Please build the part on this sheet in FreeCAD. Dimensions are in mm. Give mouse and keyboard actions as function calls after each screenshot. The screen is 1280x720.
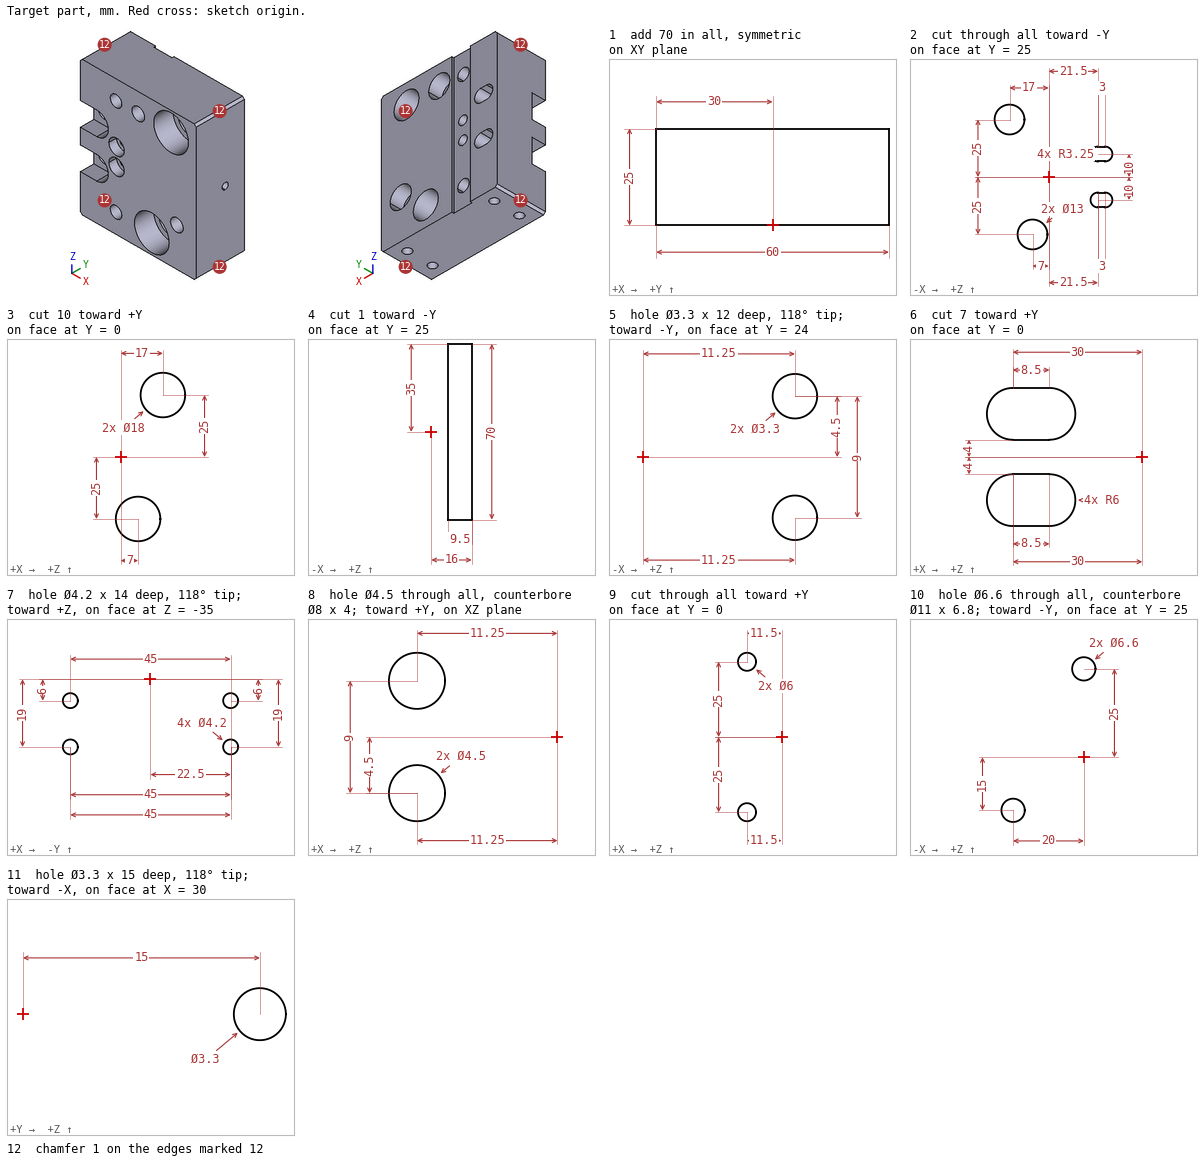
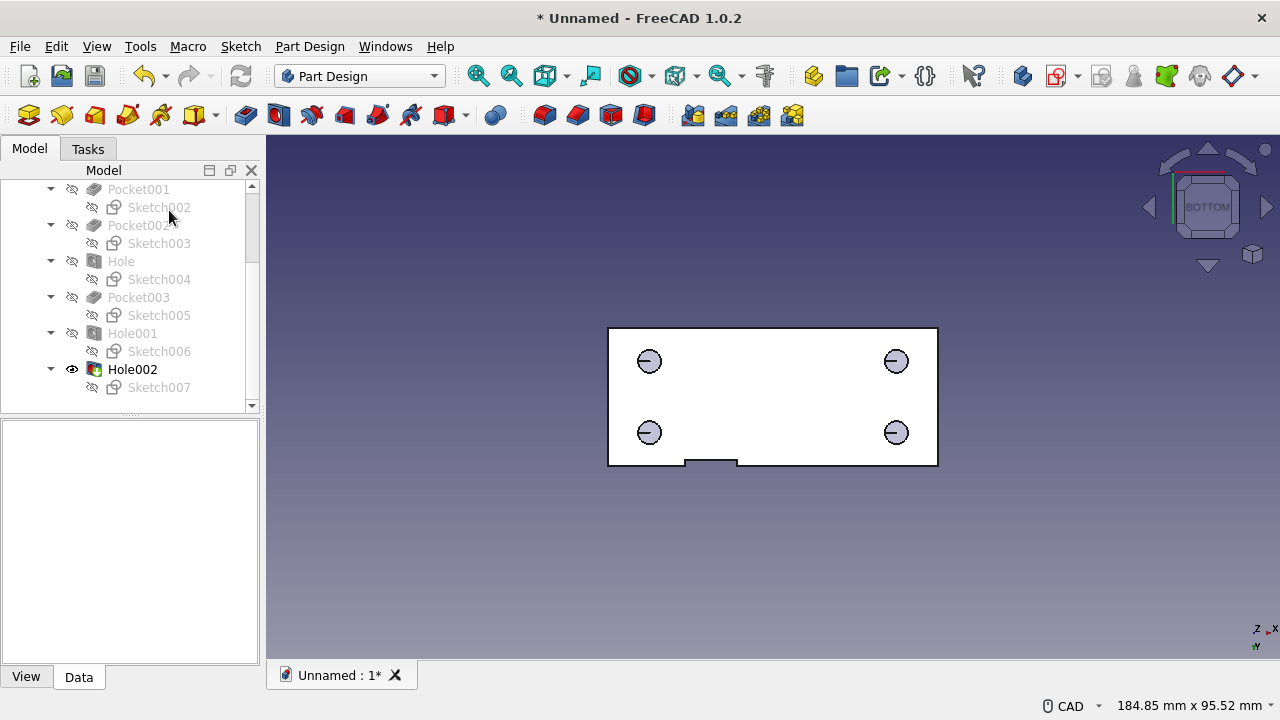
click(479, 76)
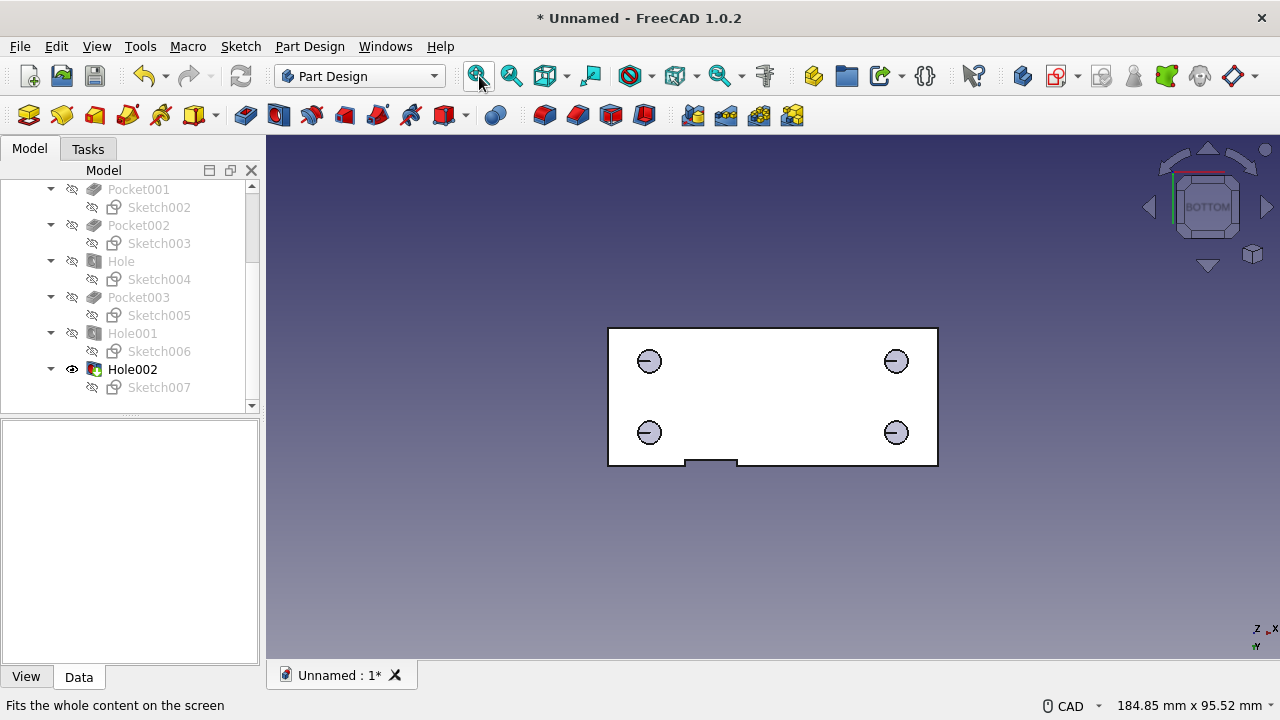
key(0)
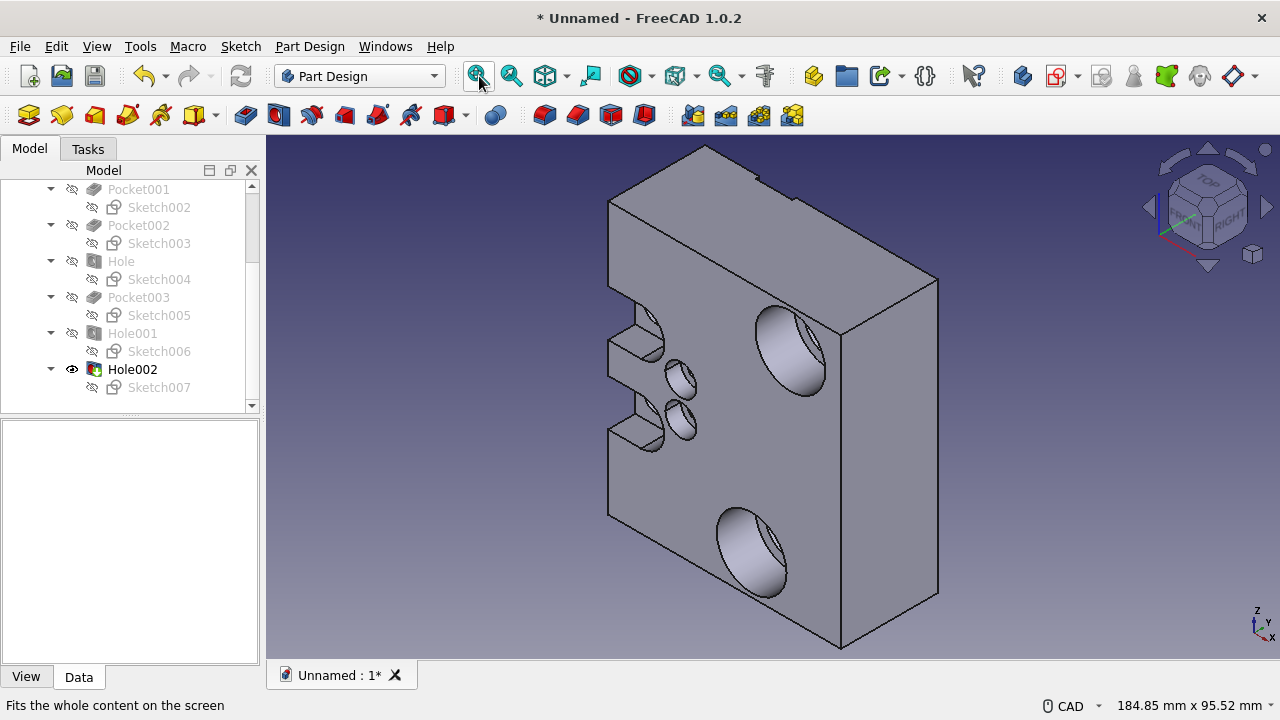
click(758, 443)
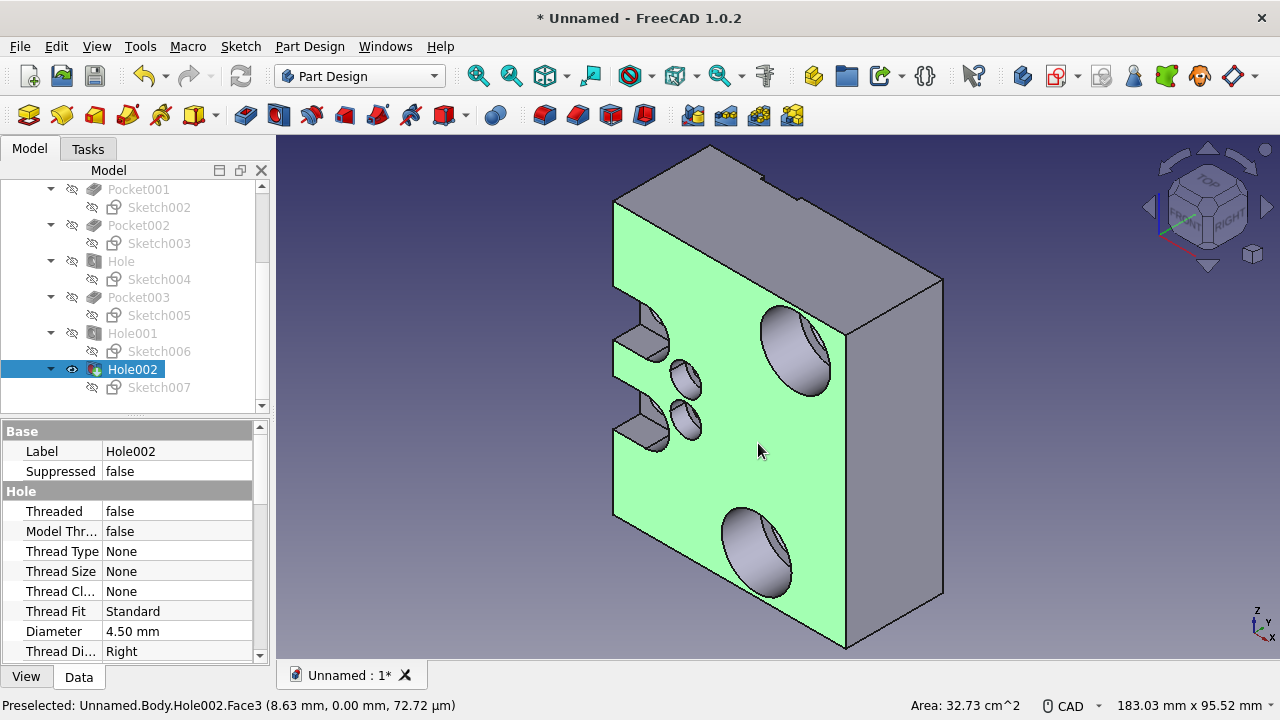
click(1056, 76)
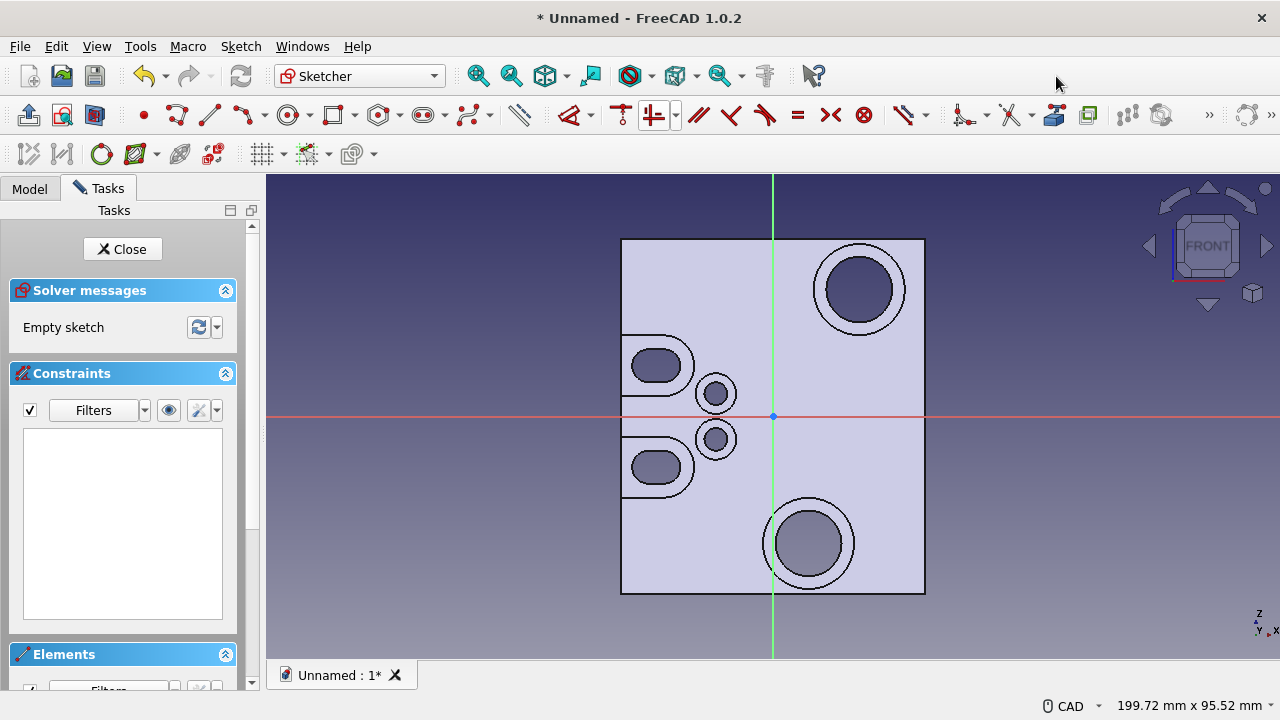
key(g)
key(c)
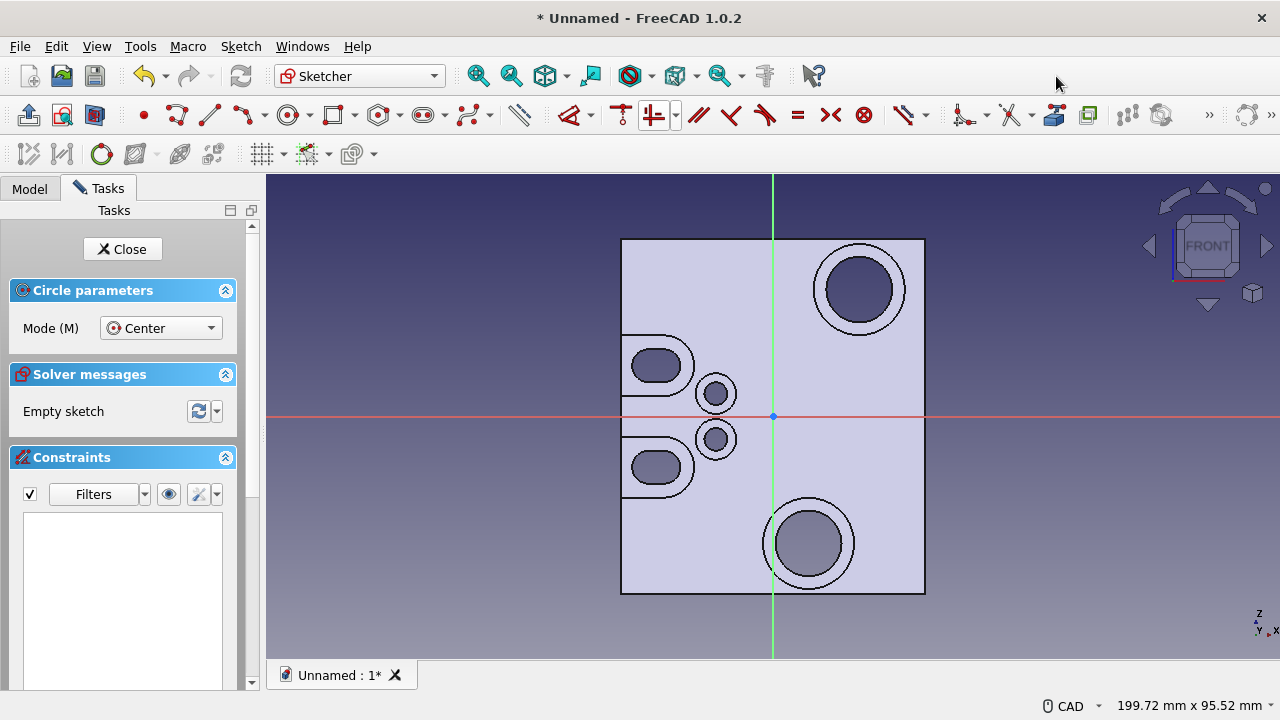
scroll(715, 290, up, 2)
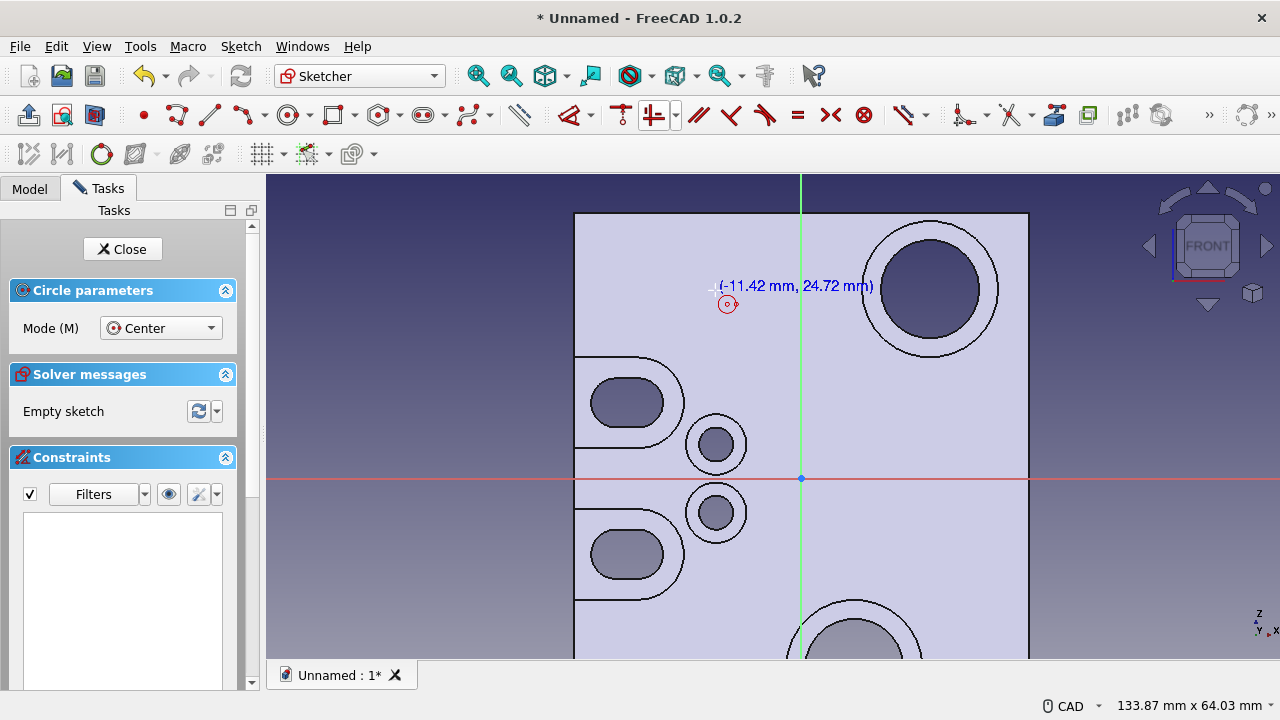
click(714, 289)
move(730, 273)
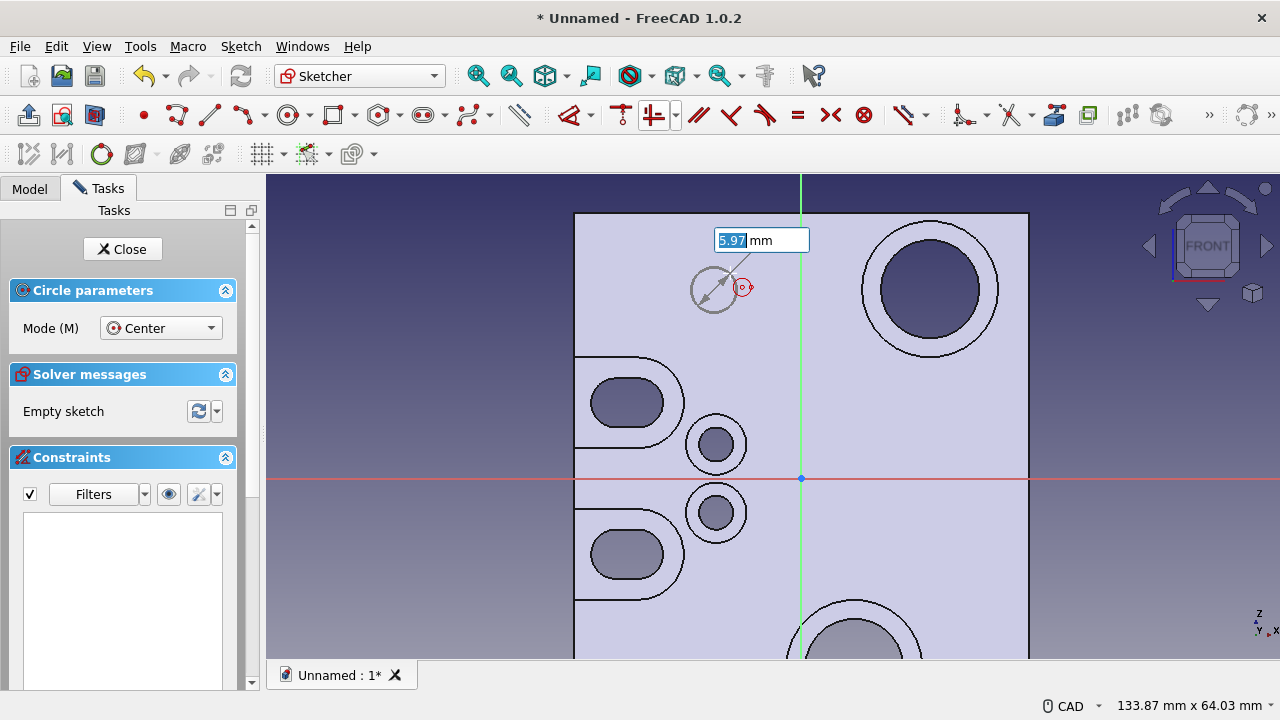
text(6)
key(Return)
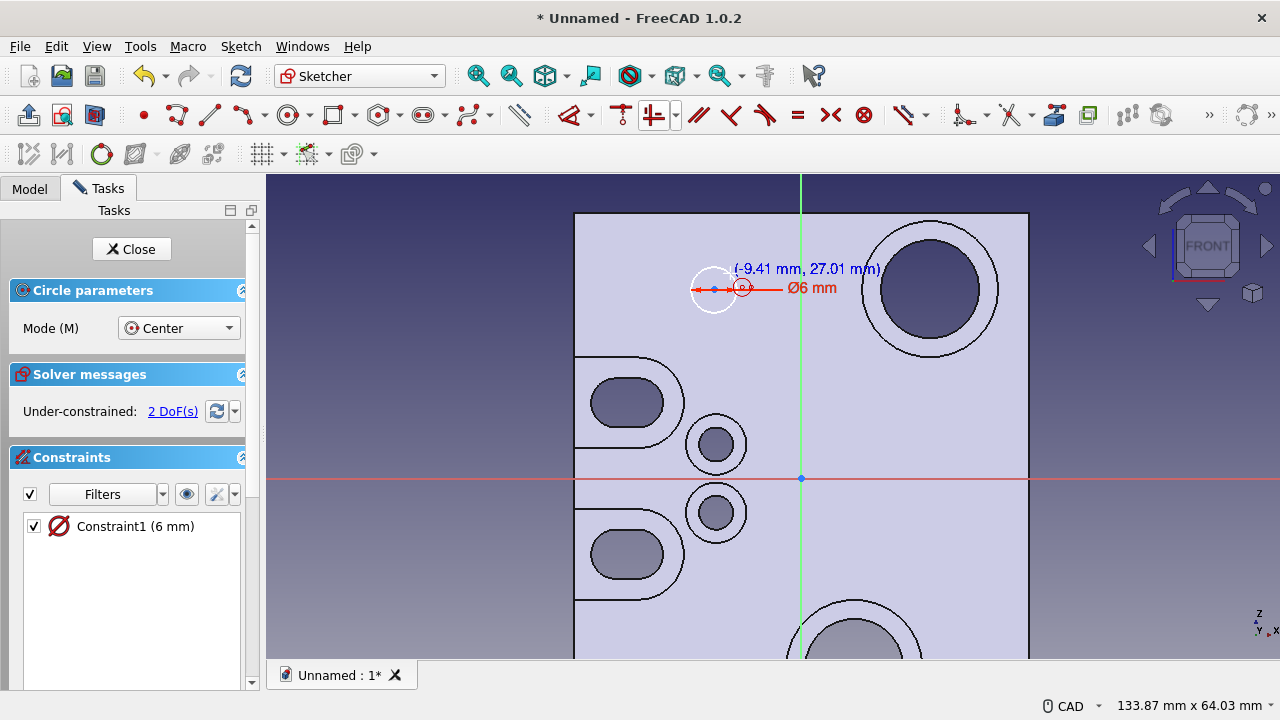
scroll(619, 290, down, 2)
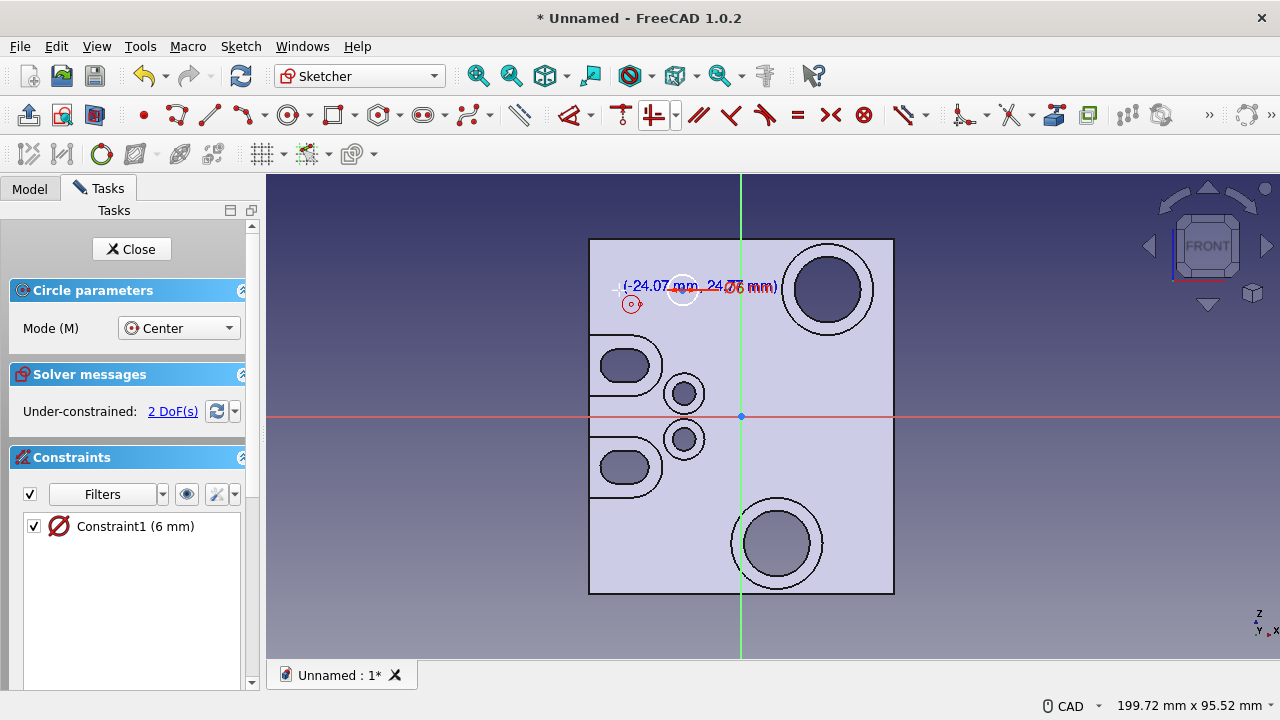
scroll(683, 543, up, 2)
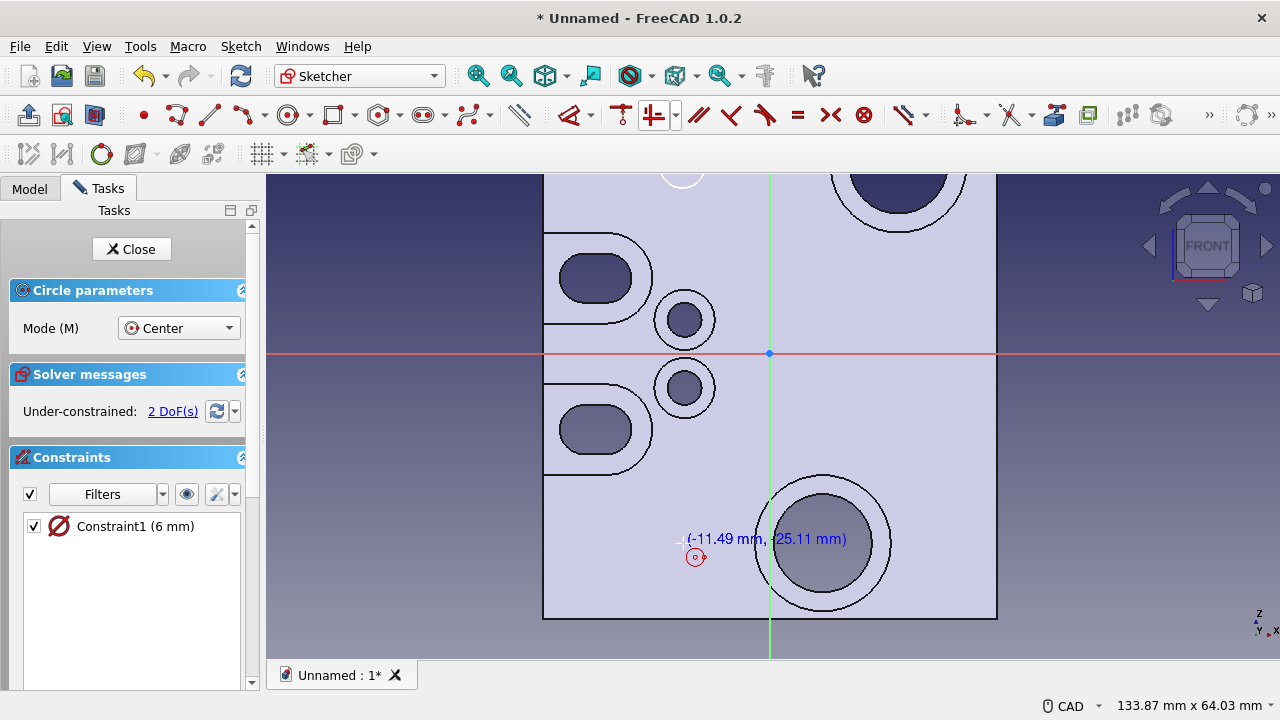
click(683, 543)
move(699, 527)